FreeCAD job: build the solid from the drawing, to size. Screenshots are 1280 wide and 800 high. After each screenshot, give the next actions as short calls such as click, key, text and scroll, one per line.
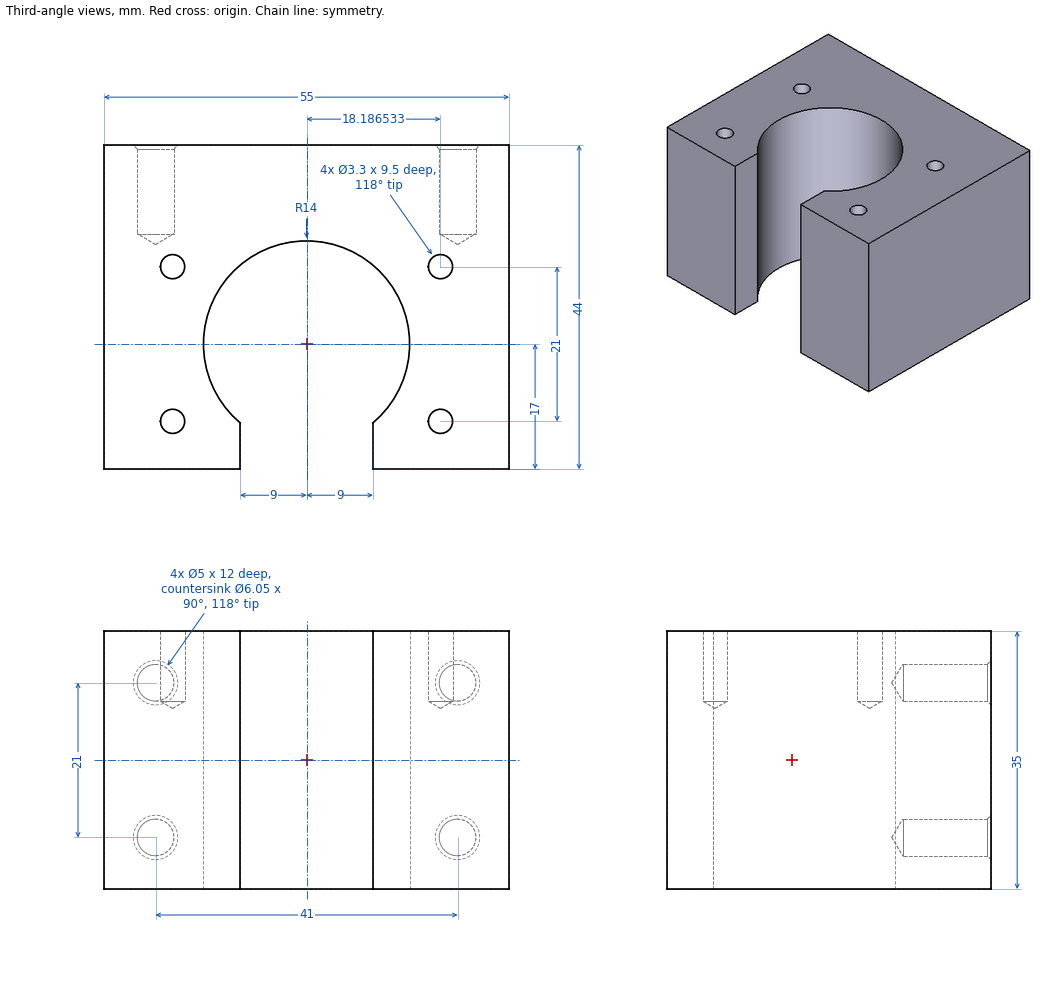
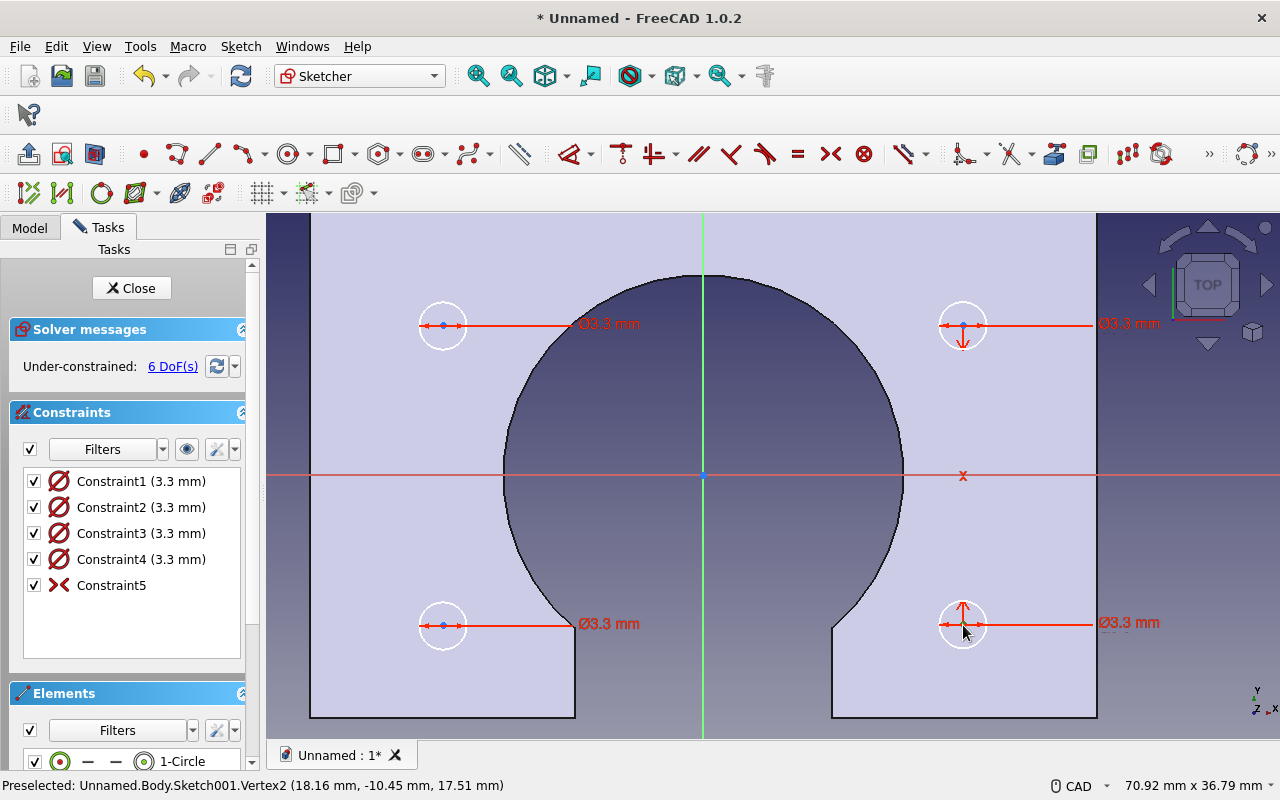
click(443, 626)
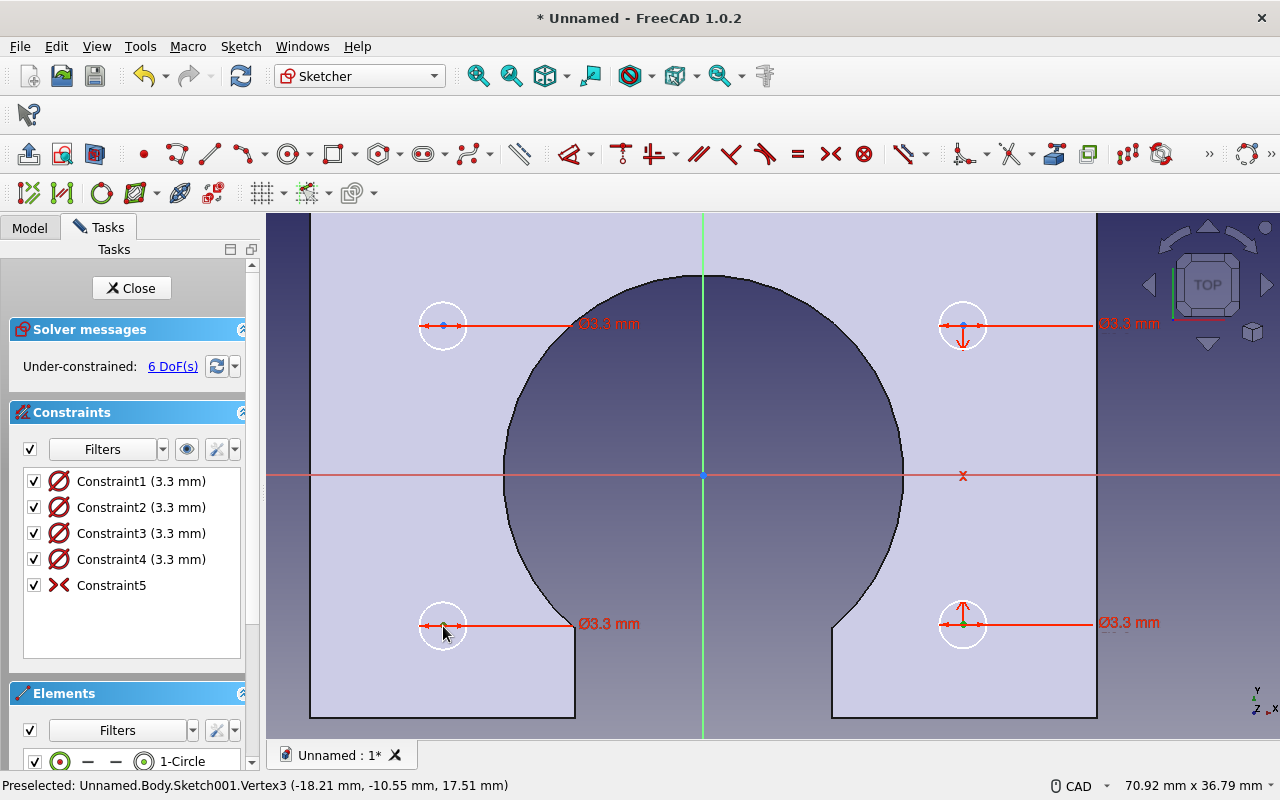
click(703, 677)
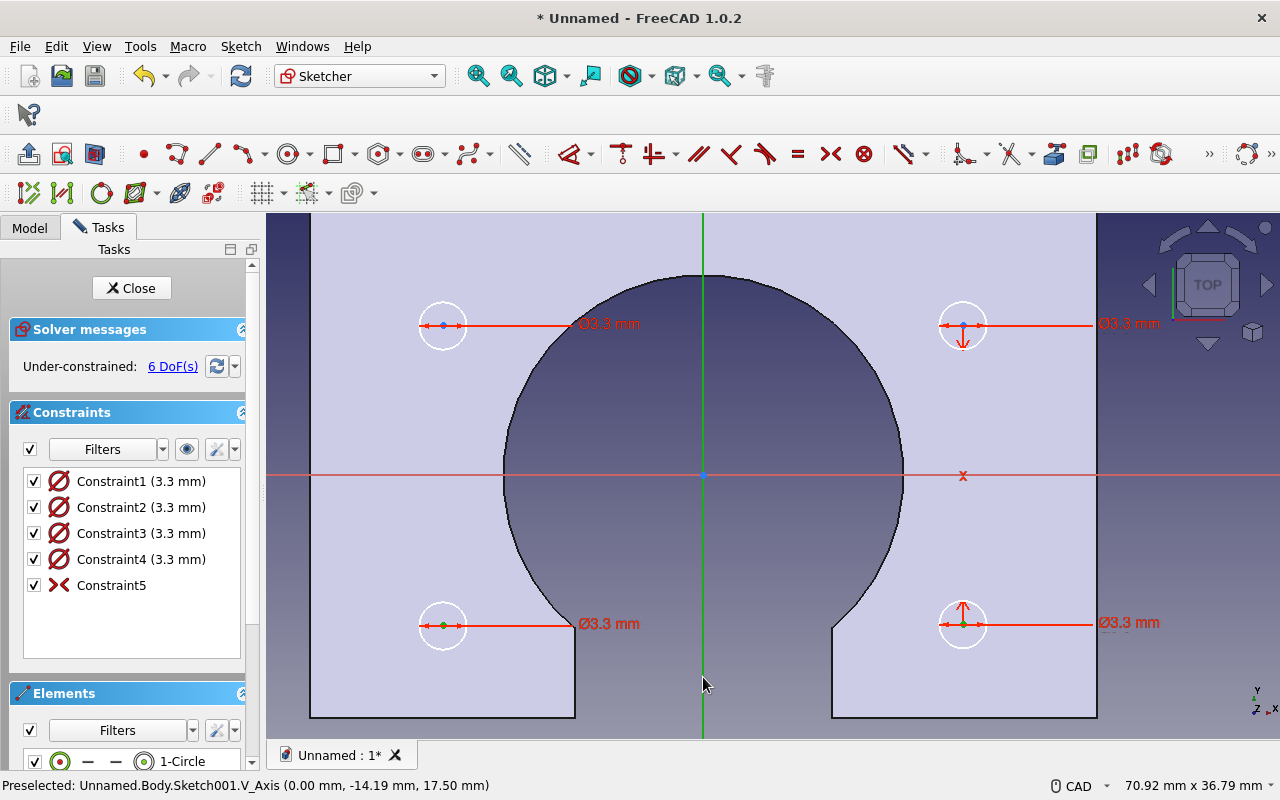
click(831, 154)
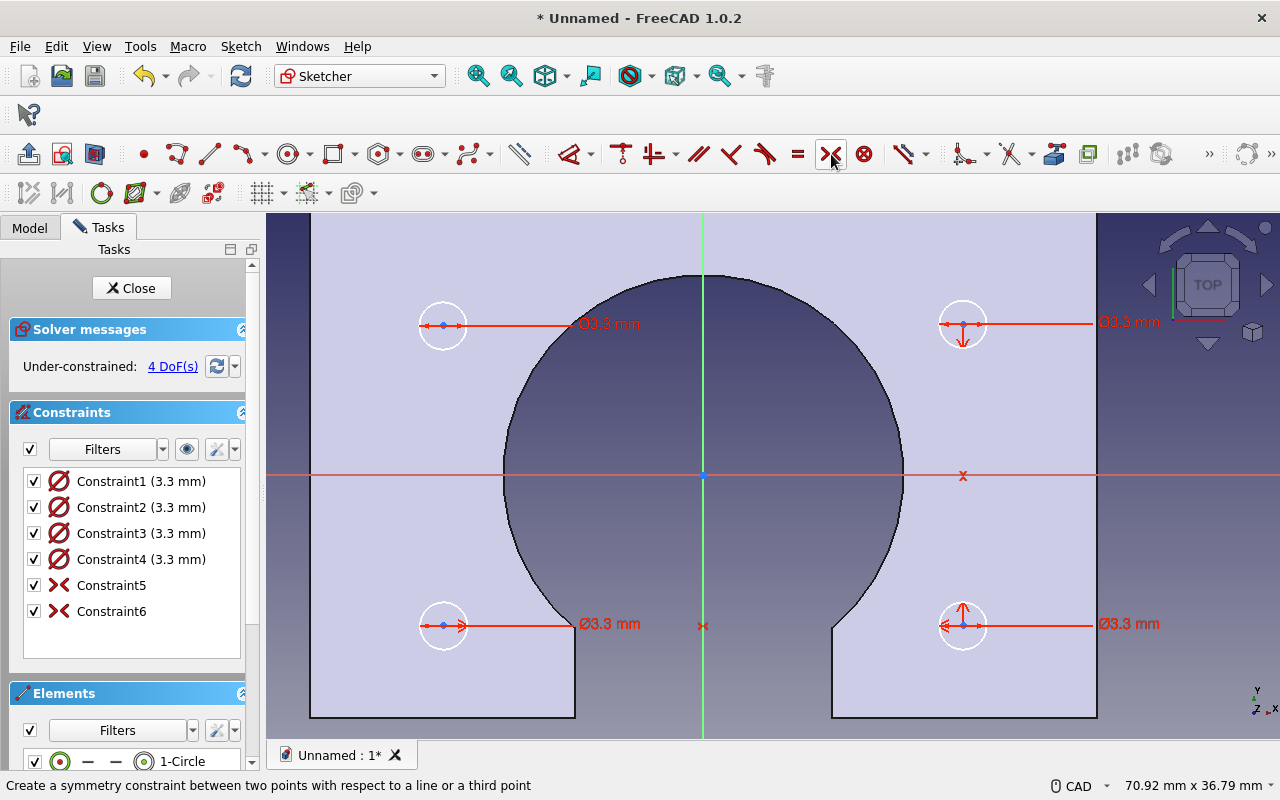
click(963, 324)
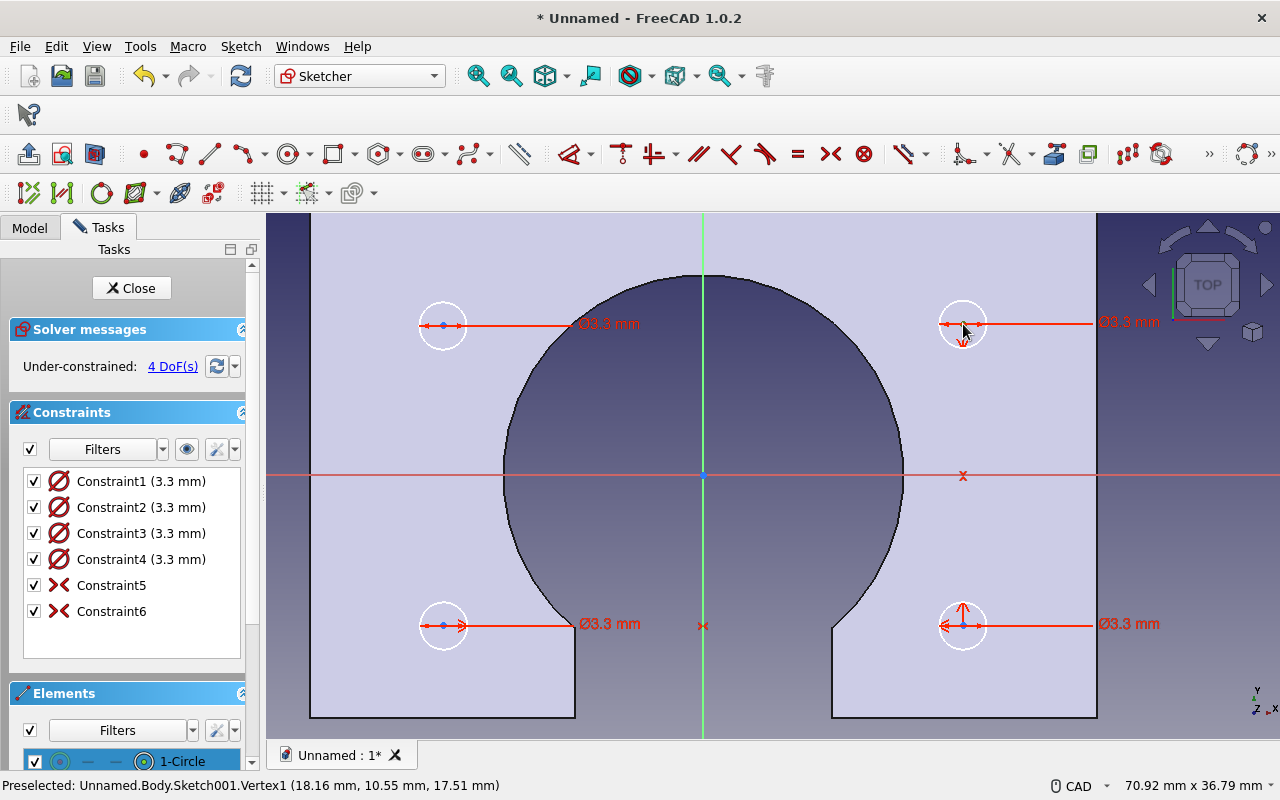
click(443, 326)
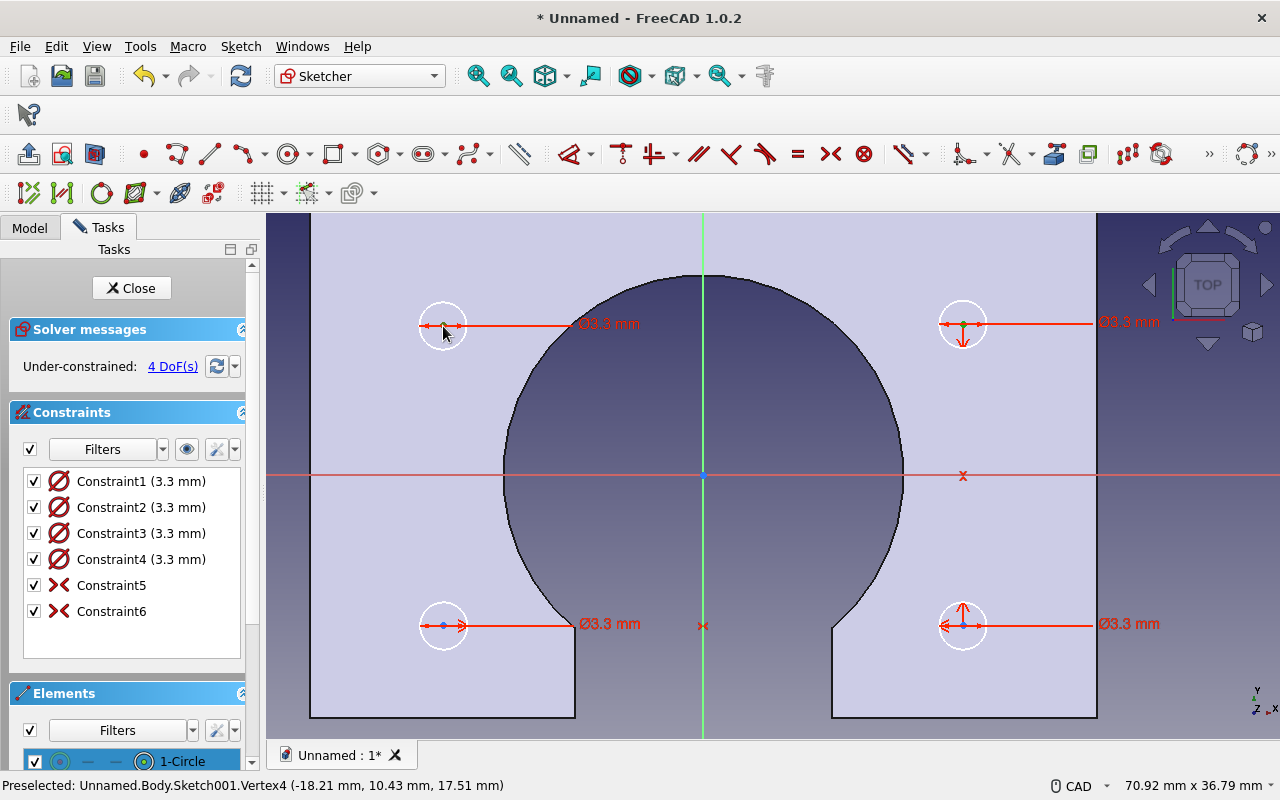
click(703, 677)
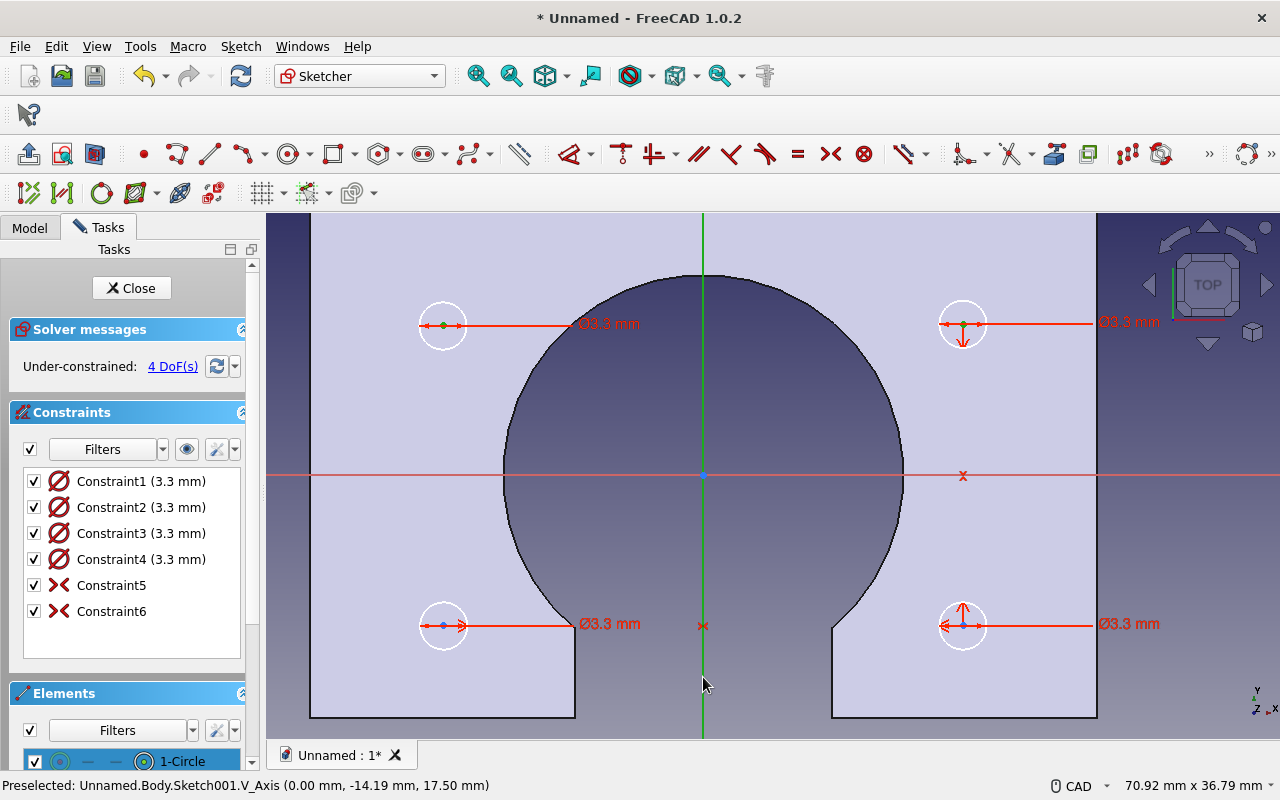
click(831, 154)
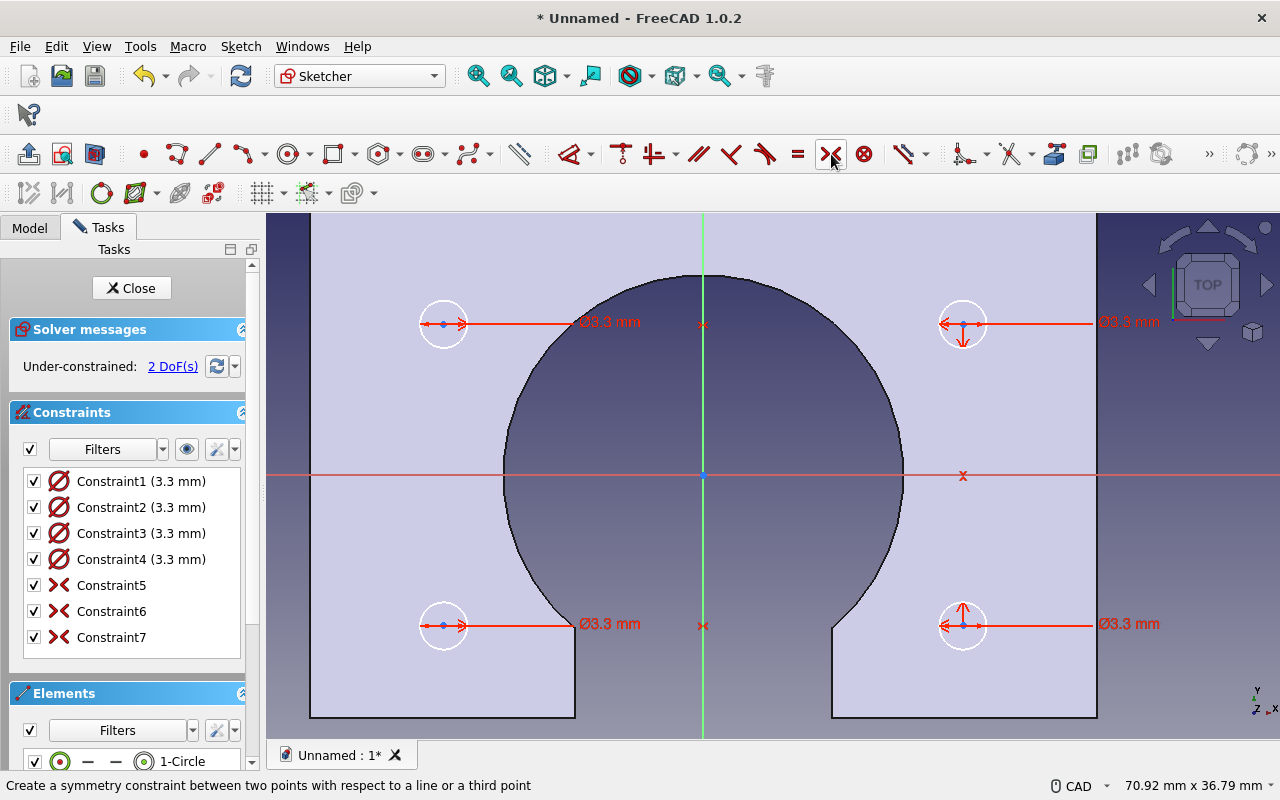
click(568, 154)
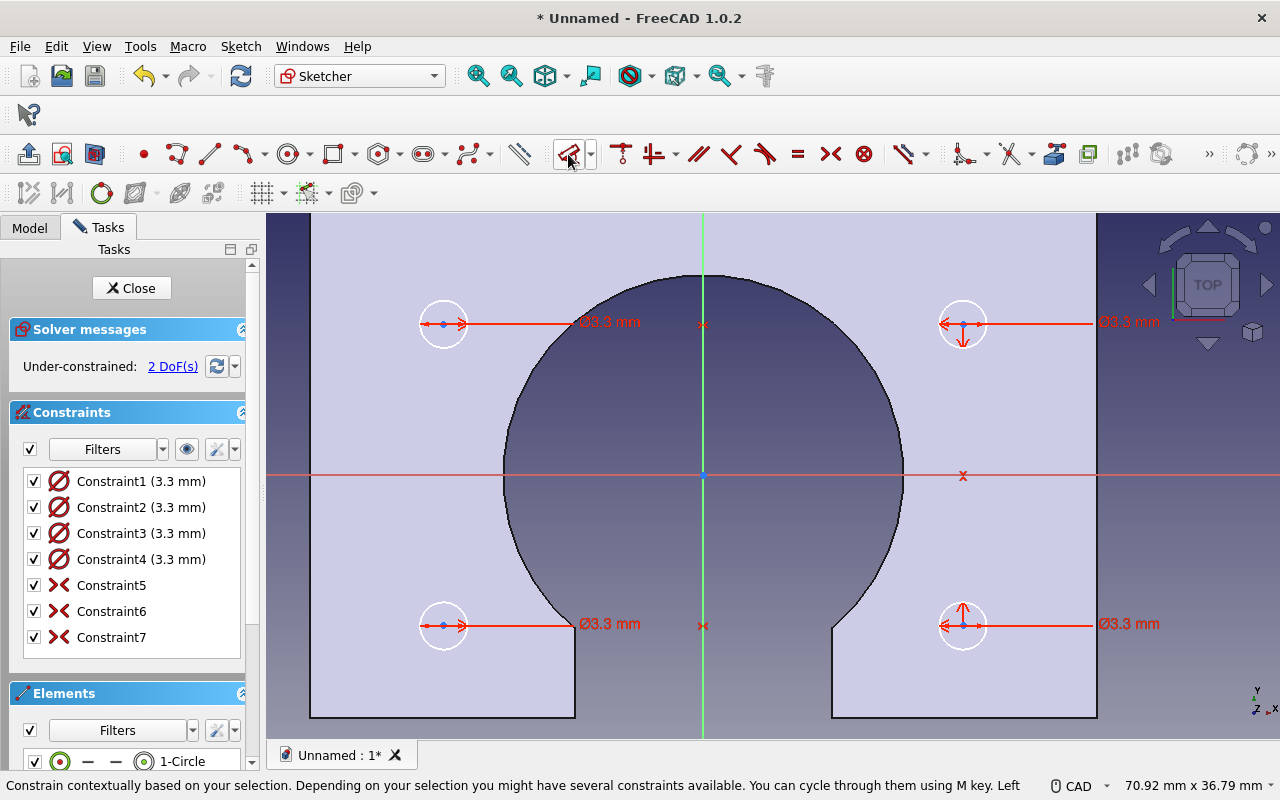
click(963, 324)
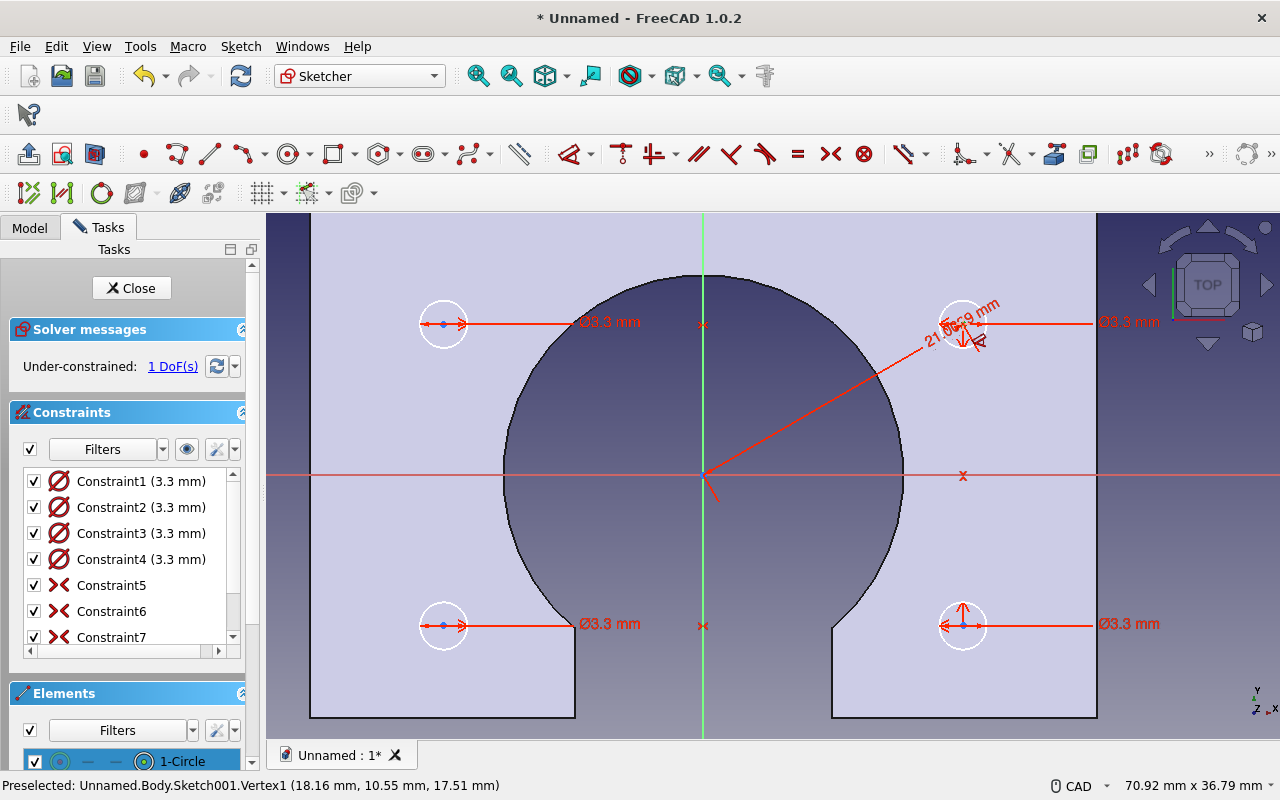
click(963, 626)
click(997, 406)